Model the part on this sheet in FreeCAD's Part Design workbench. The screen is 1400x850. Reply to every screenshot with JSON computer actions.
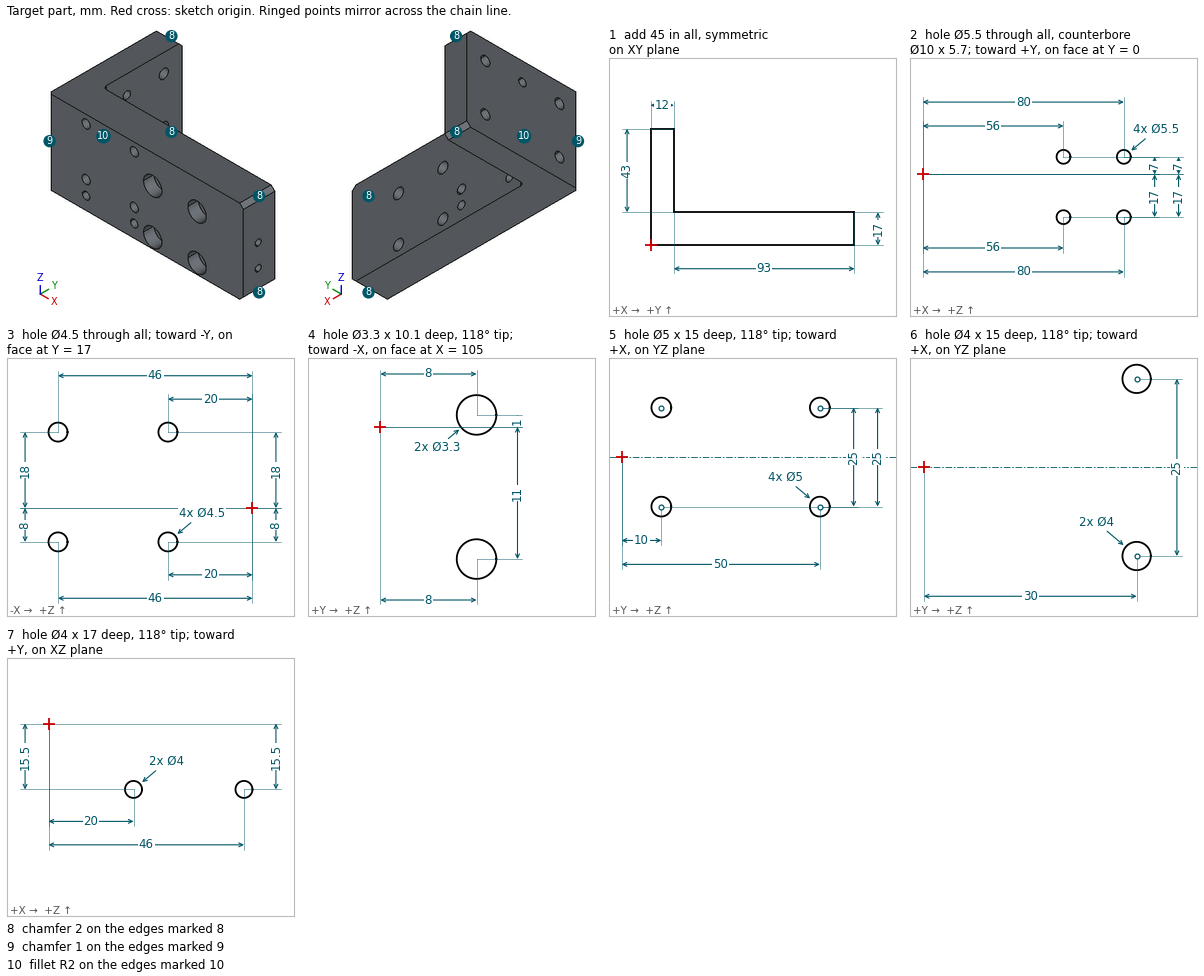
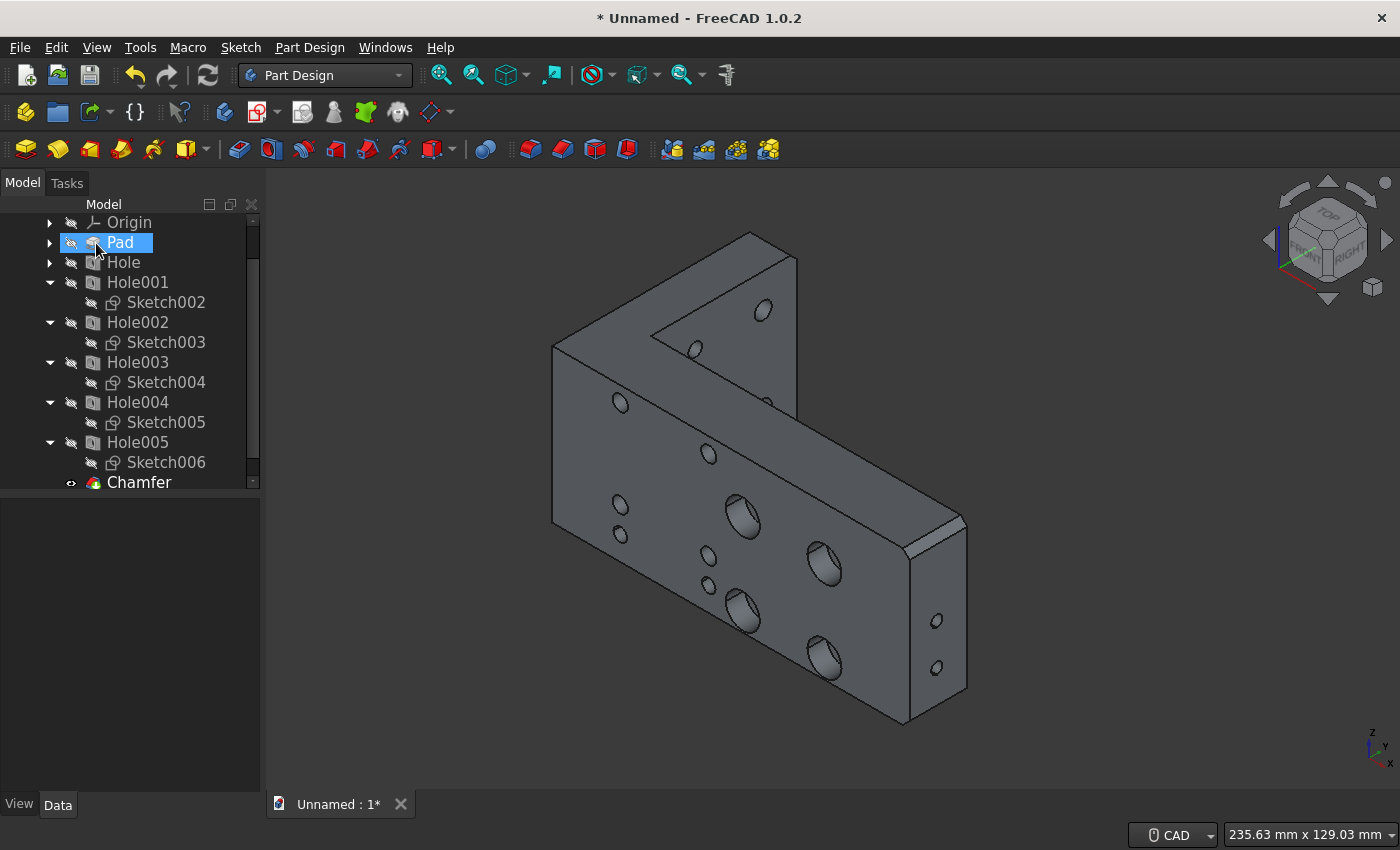
{"action": "key", "text": "2"}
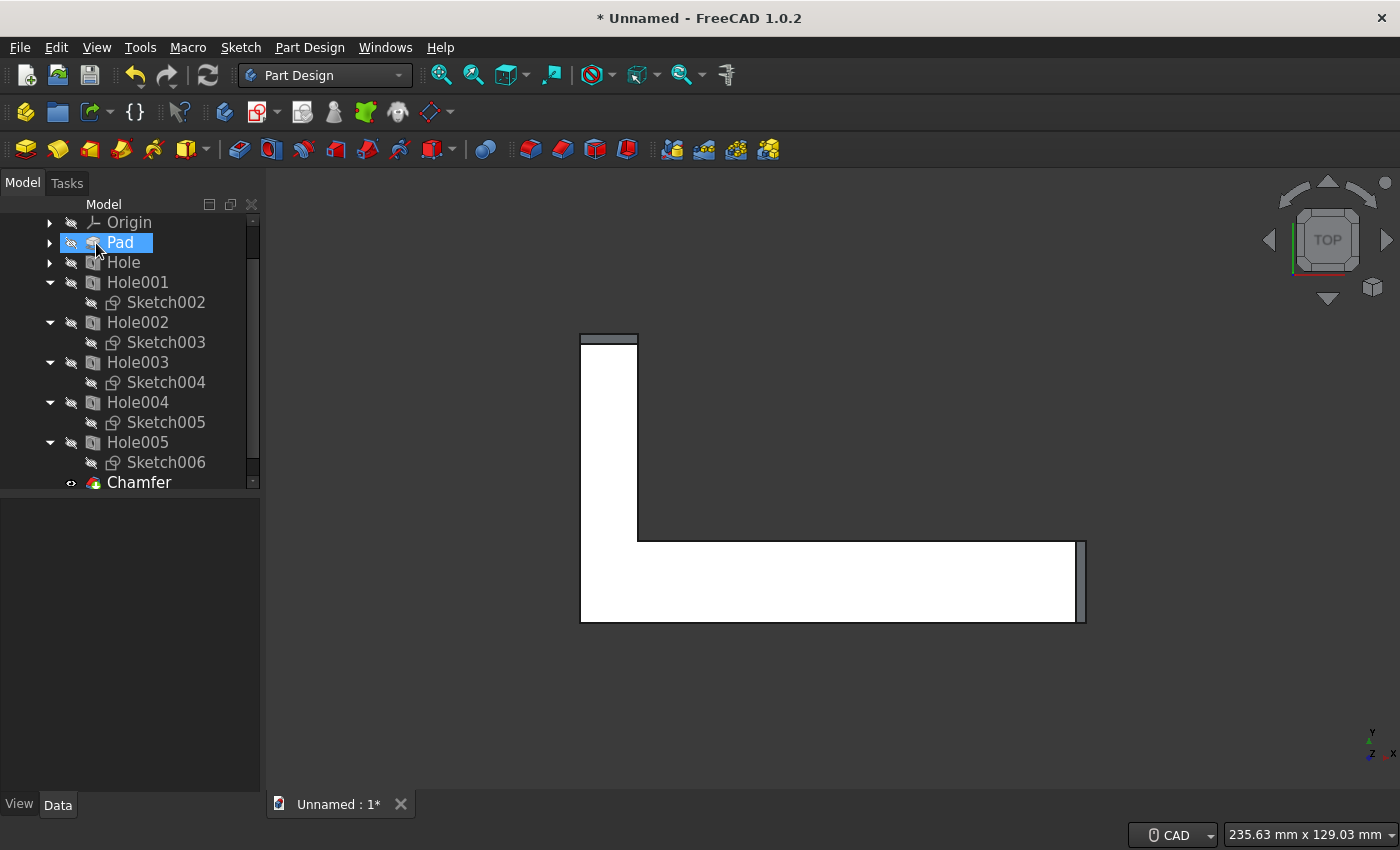
{"action": "key", "text": "1"}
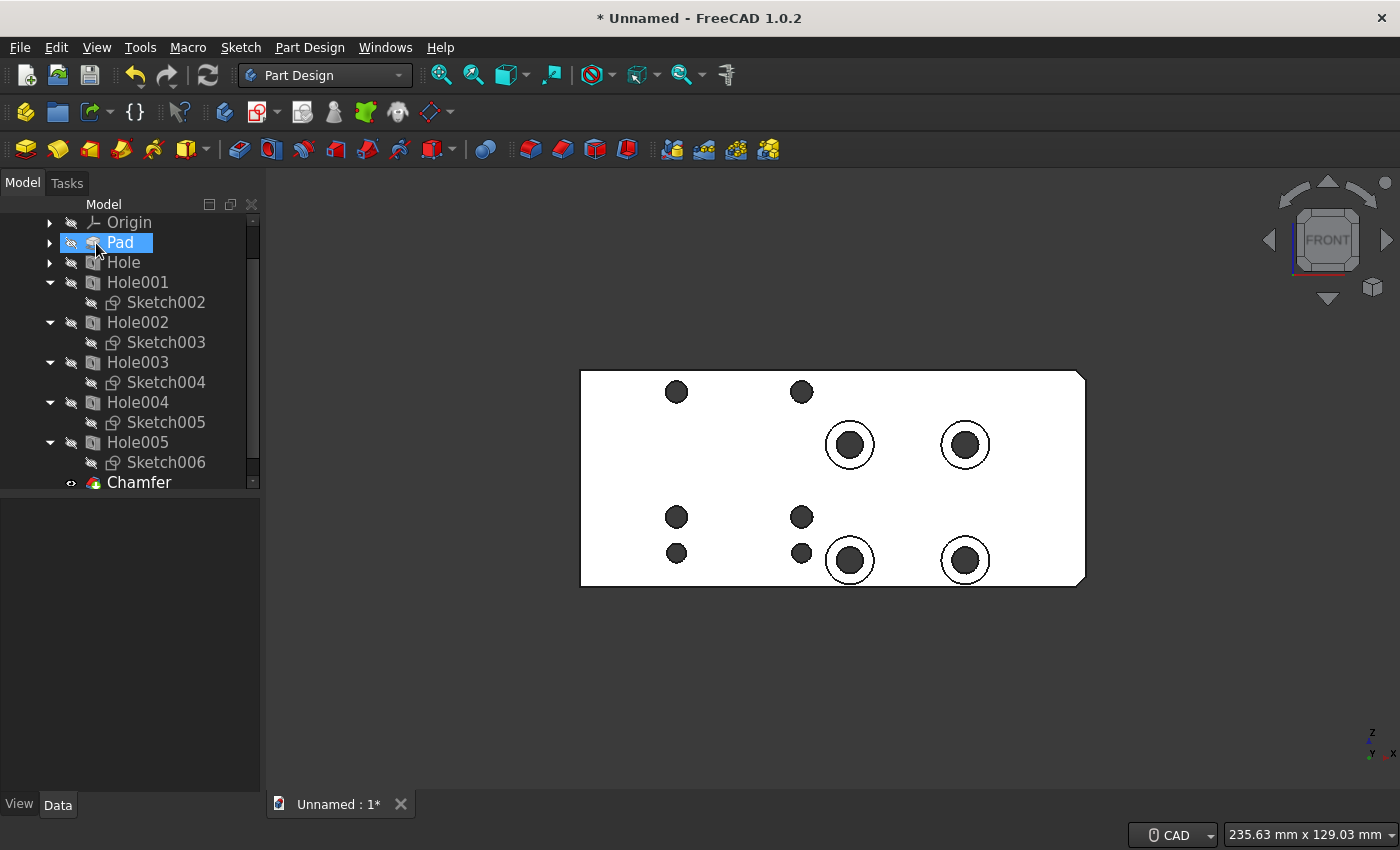
{"action": "key", "text": "v f"}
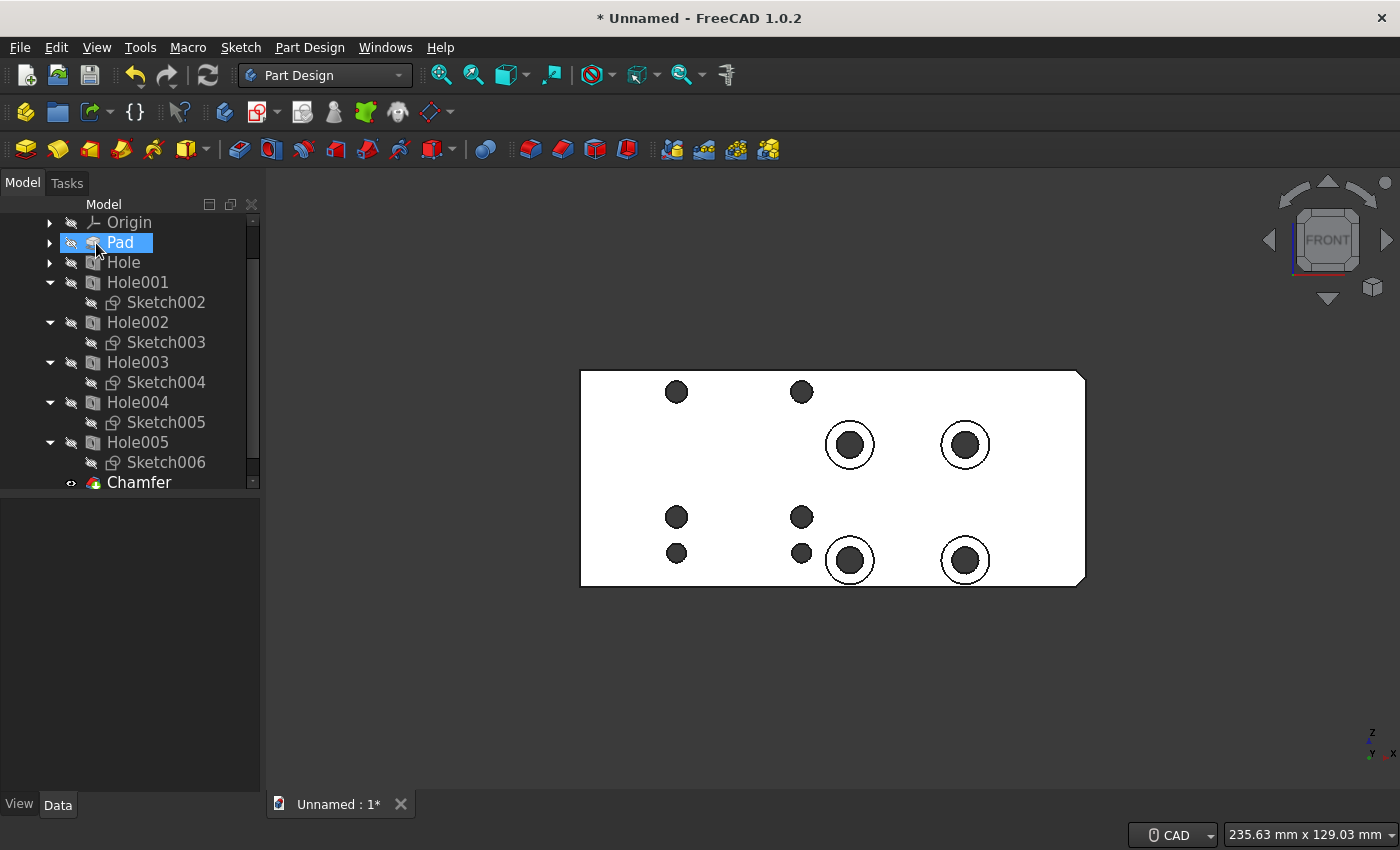
{"action": "left_click", "coordinate": [580, 478]}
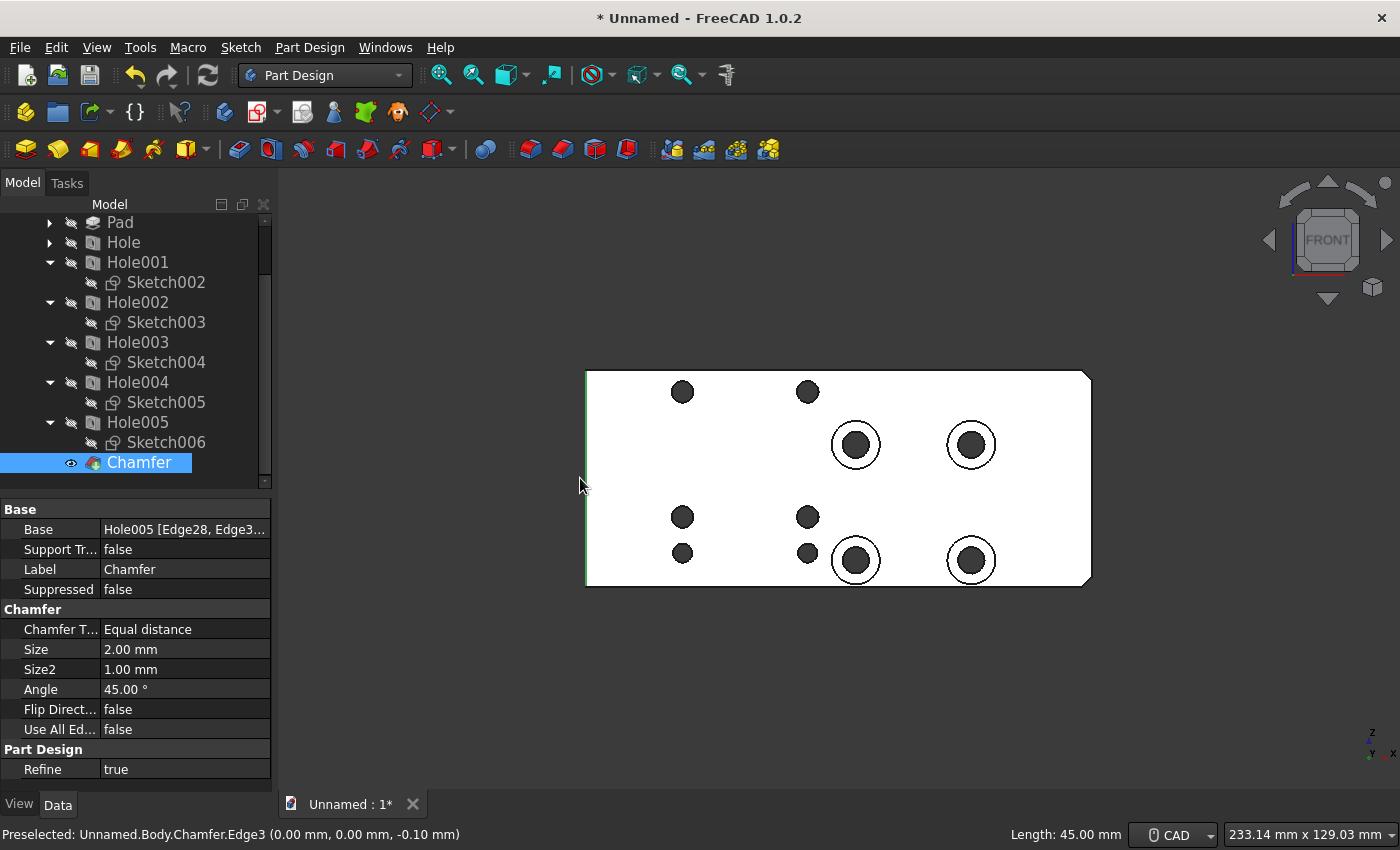
{"action": "left_click", "coordinate": [564, 150]}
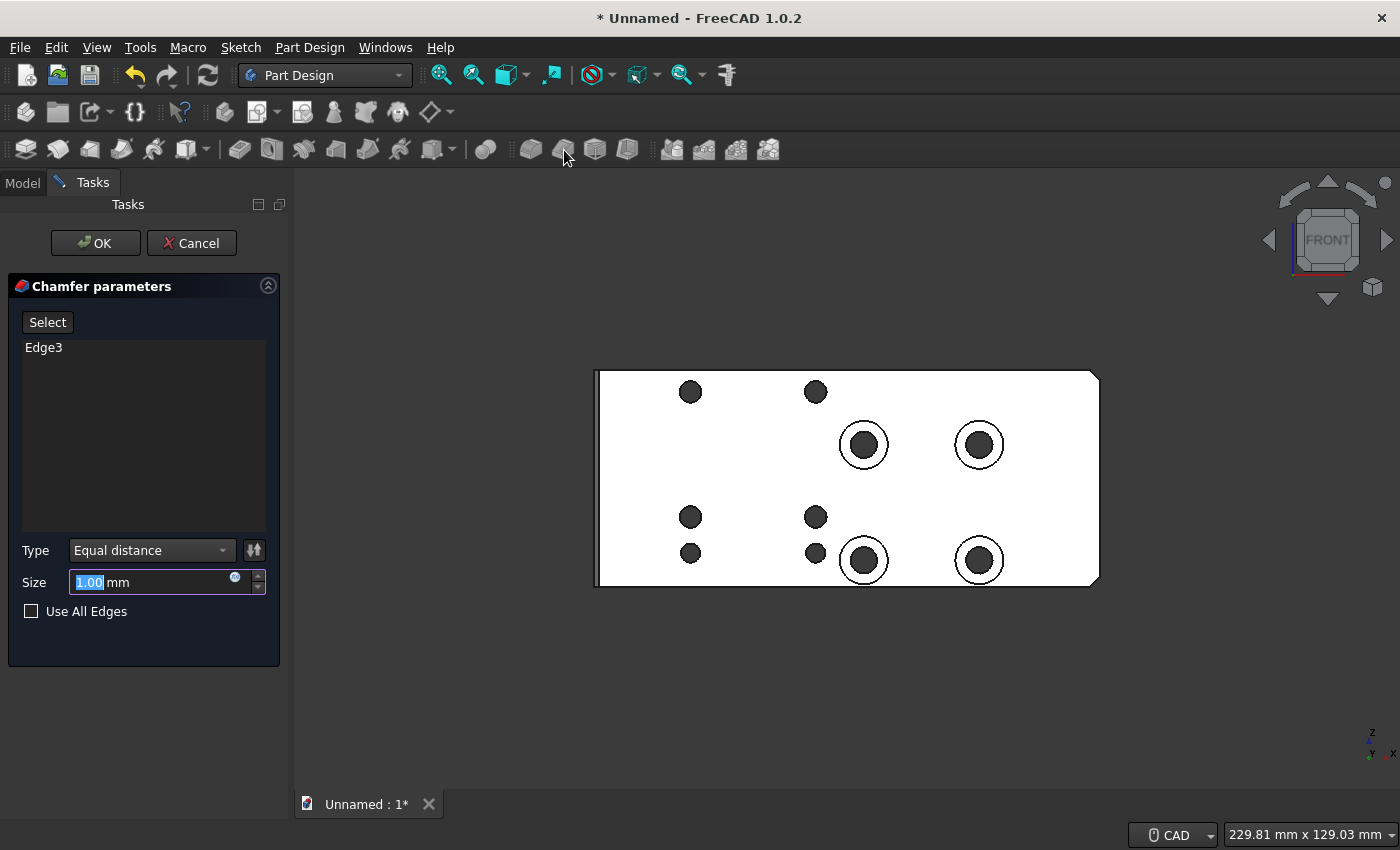
{"action": "type", "text": "1"}
{"action": "key", "text": "Tab"}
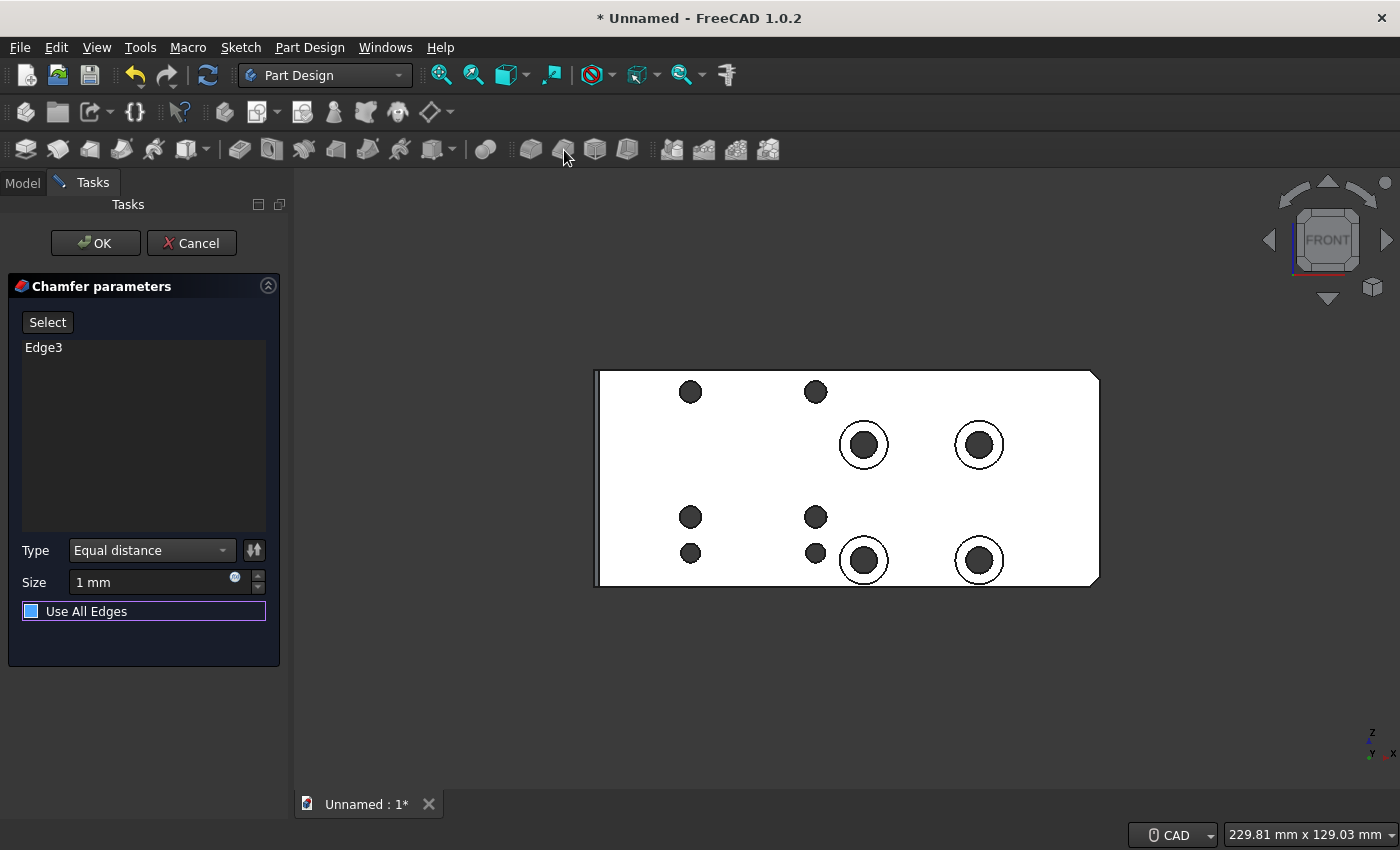
{"action": "left_click", "coordinate": [96, 243]}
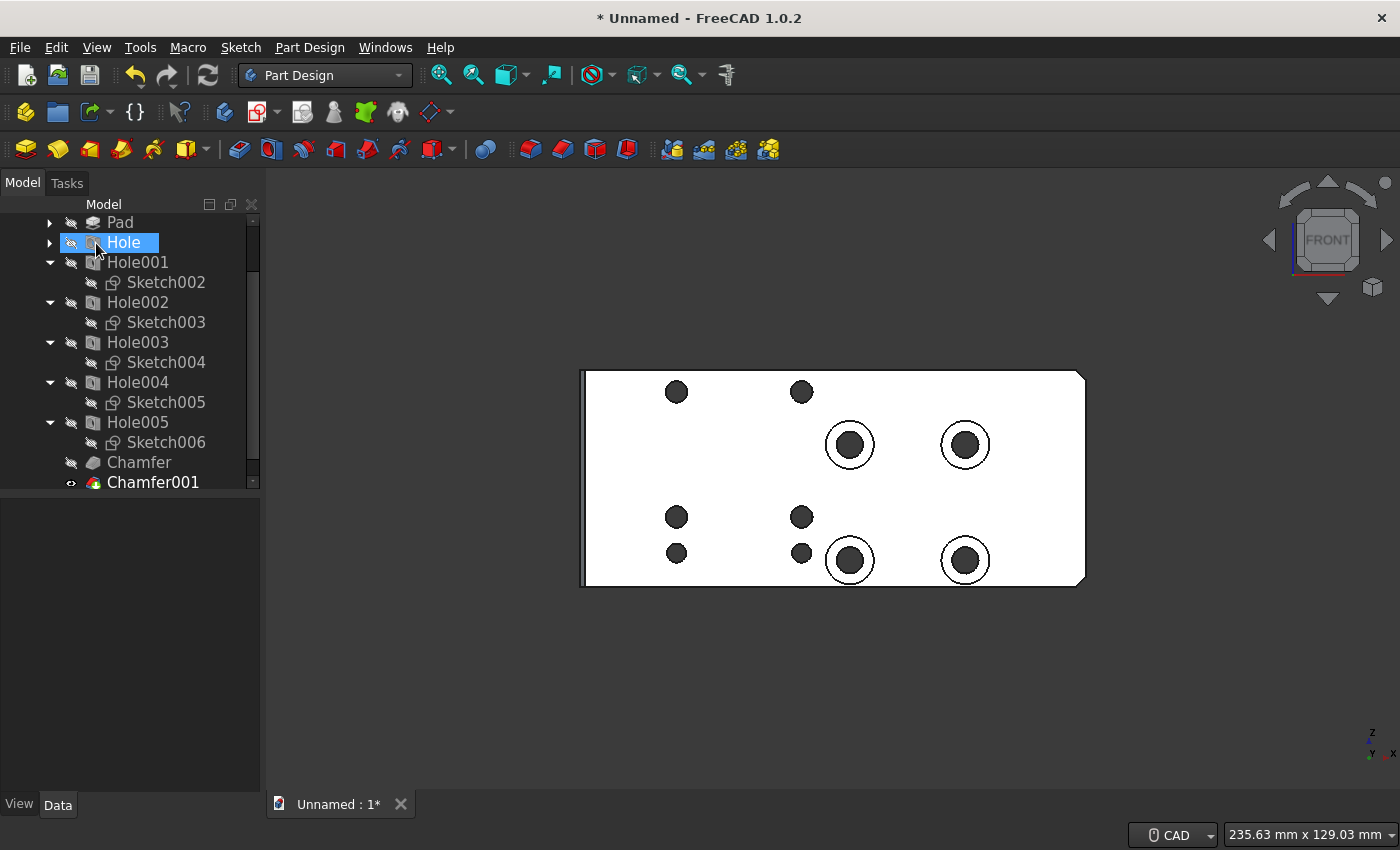
{"action": "key", "text": "v f"}